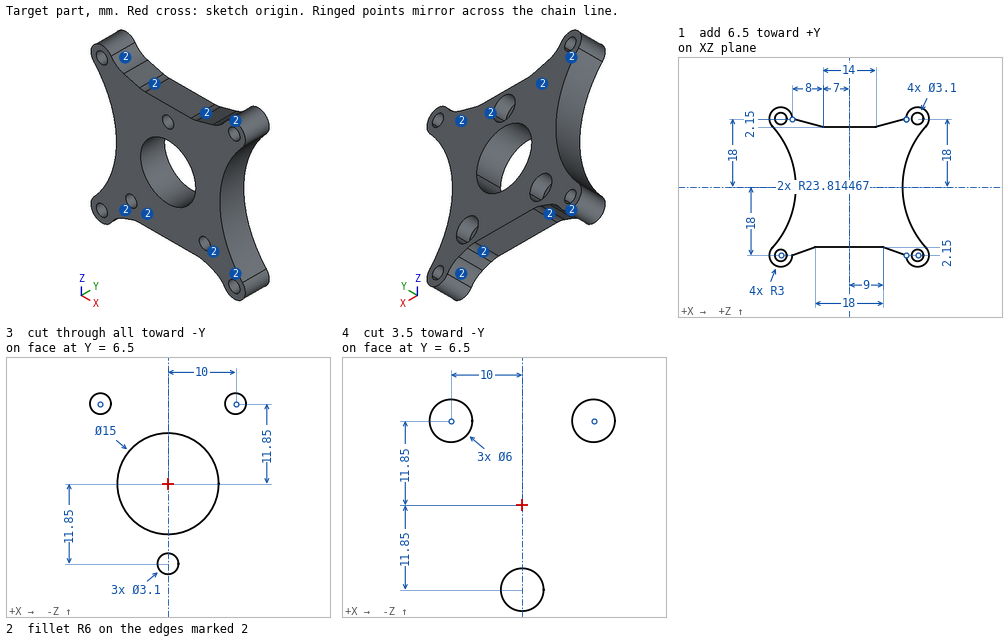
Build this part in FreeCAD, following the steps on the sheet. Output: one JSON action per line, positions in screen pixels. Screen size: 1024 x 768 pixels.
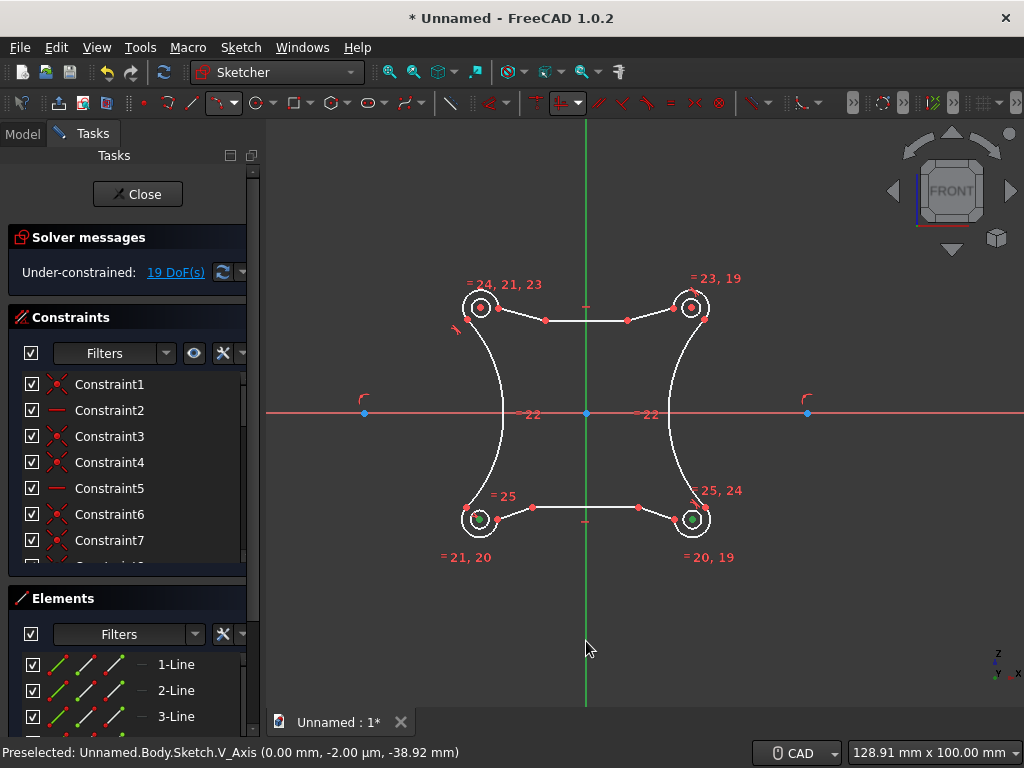
{"action": "left_click", "coordinate": [696, 104]}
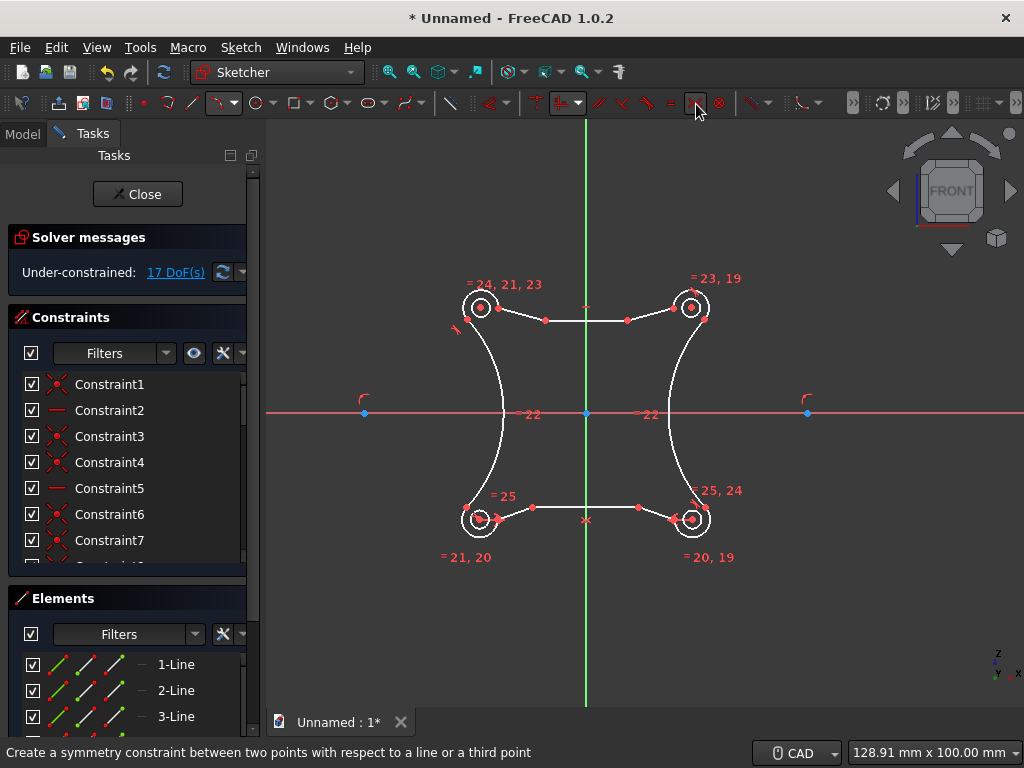
{"action": "left_click", "coordinate": [499, 308]}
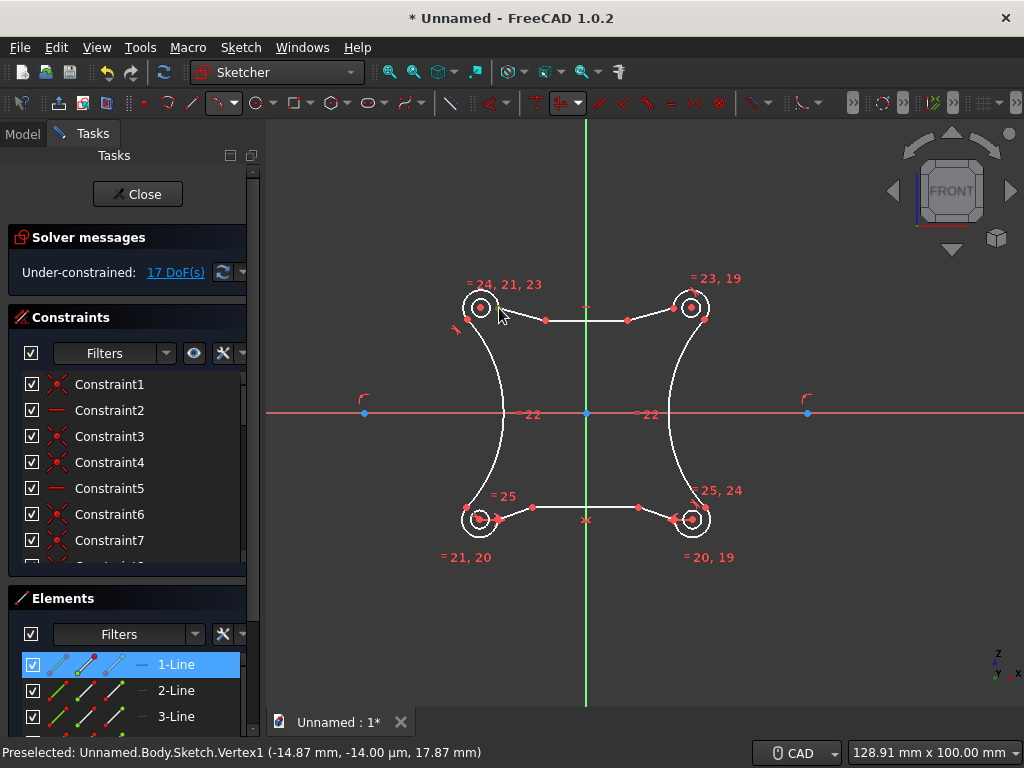
{"action": "left_click", "coordinate": [674, 308]}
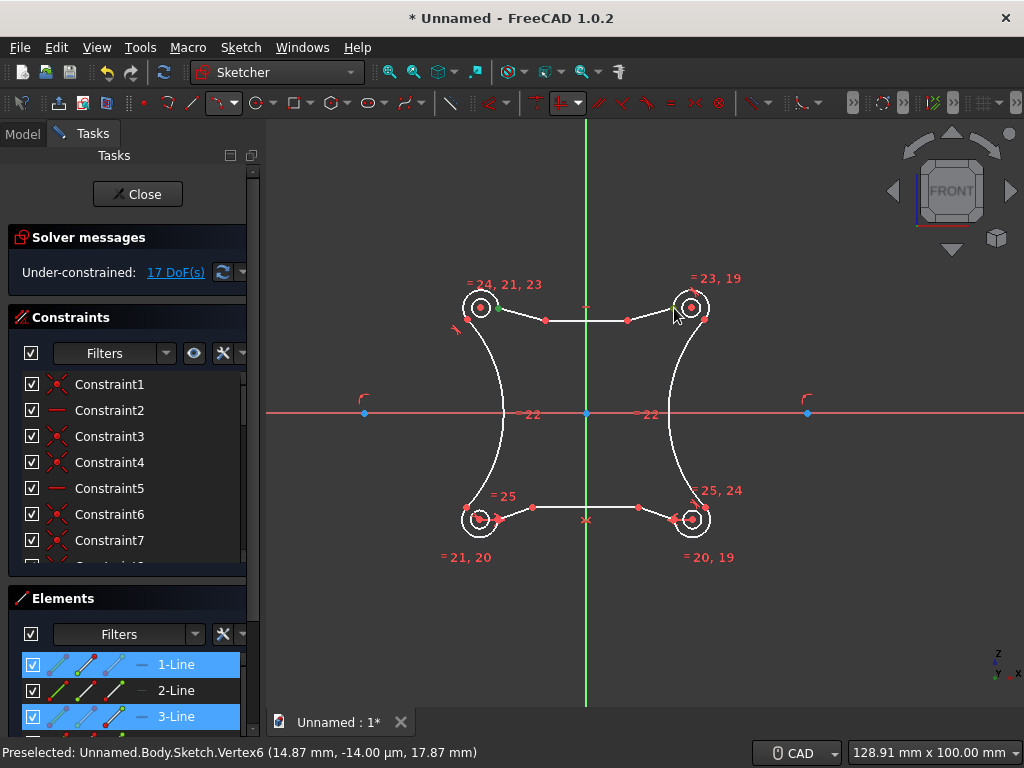
{"action": "left_click", "coordinate": [586, 641]}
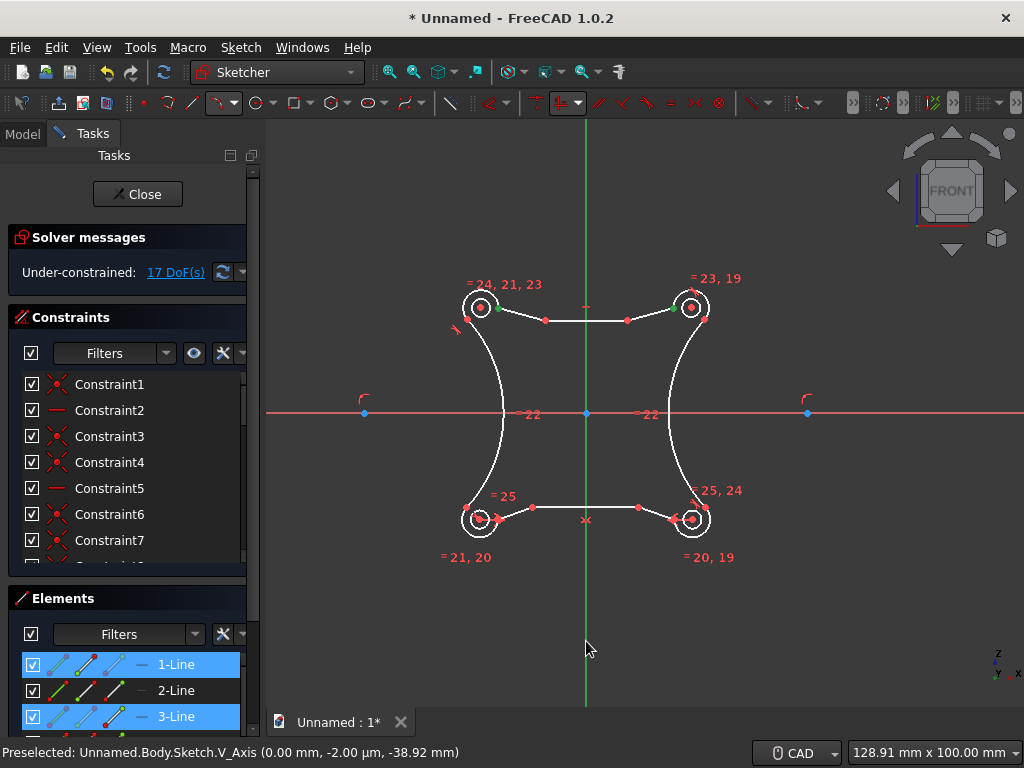
{"action": "left_click", "coordinate": [696, 104]}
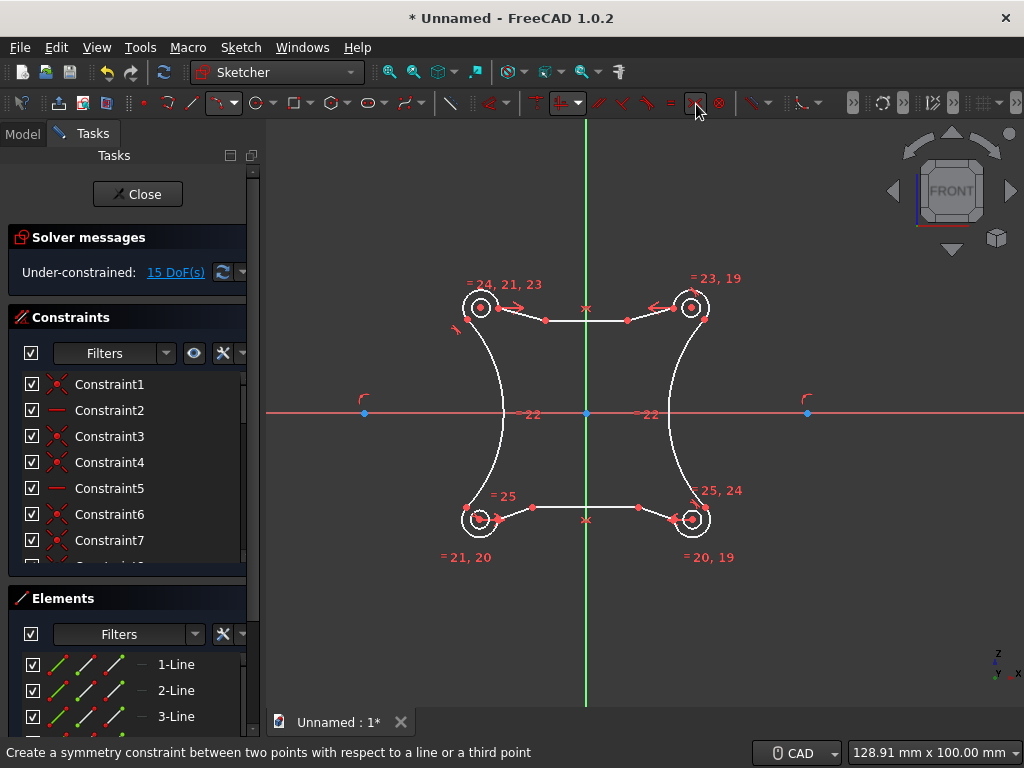
{"action": "left_click", "coordinate": [674, 308]}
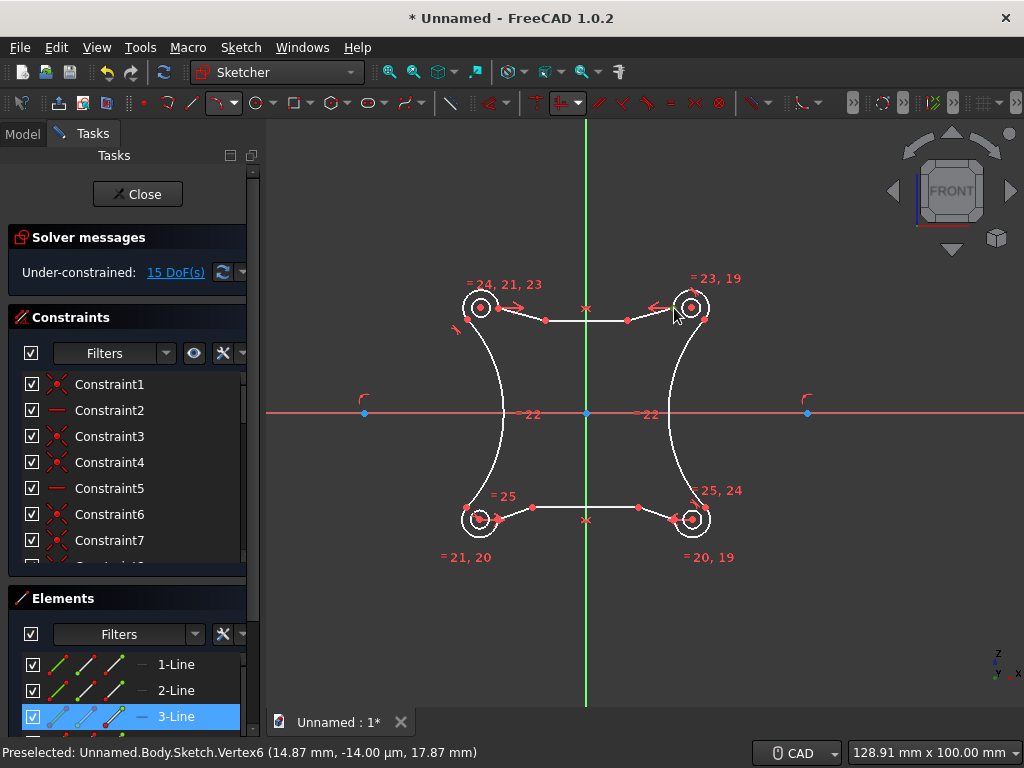
{"action": "left_click", "coordinate": [675, 520]}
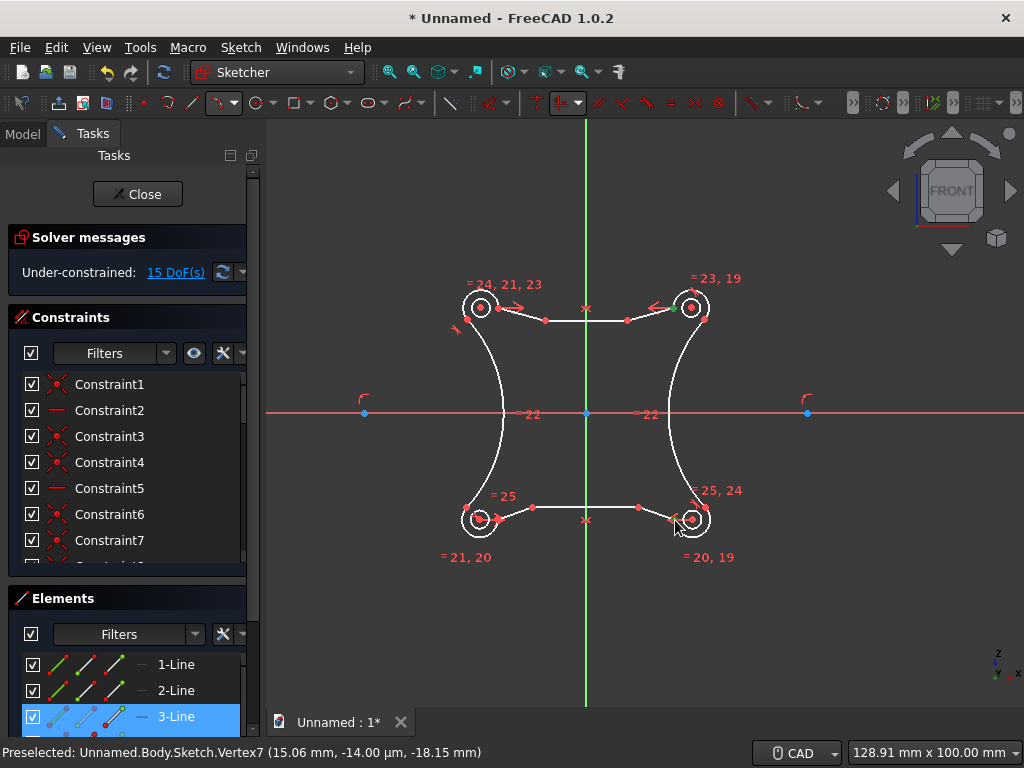
{"action": "left_click", "coordinate": [334, 413]}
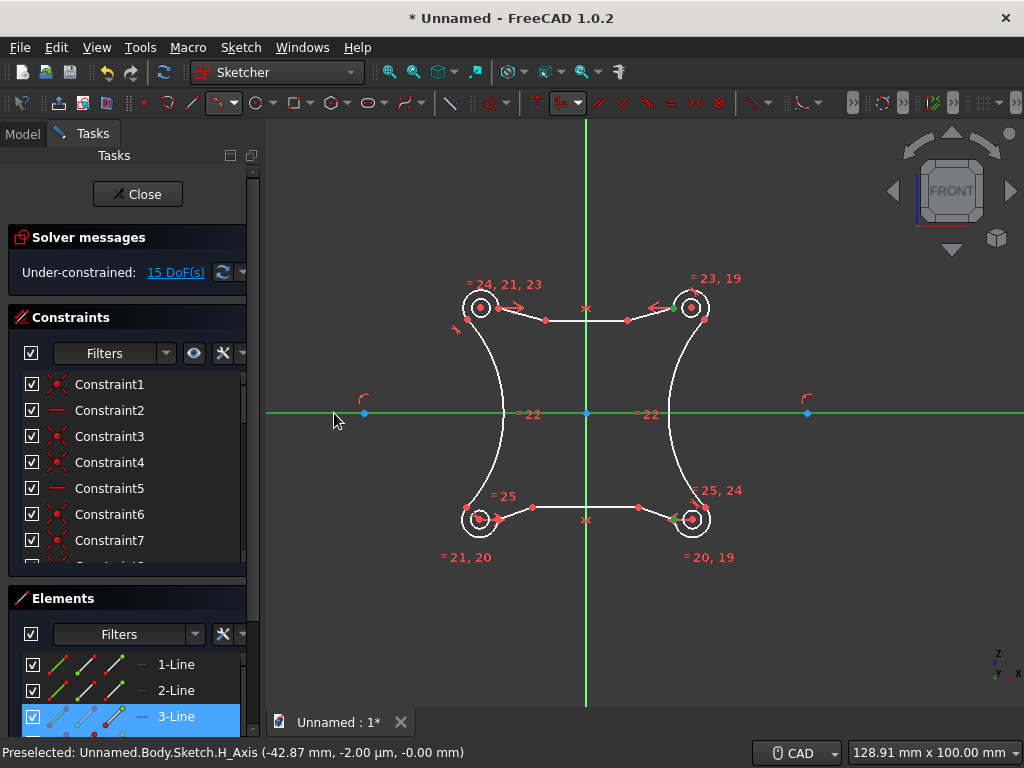
{"action": "left_click", "coordinate": [696, 104]}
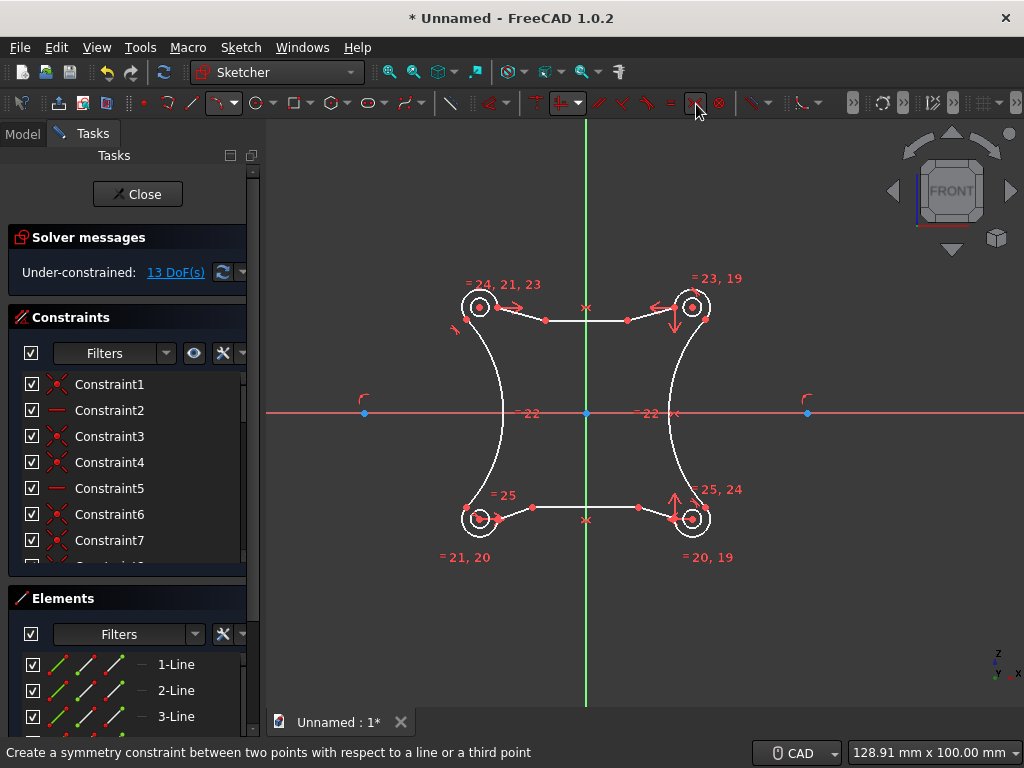
{"action": "scroll", "coordinate": [708, 300], "scroll_direction": "up", "scroll_amount": 5}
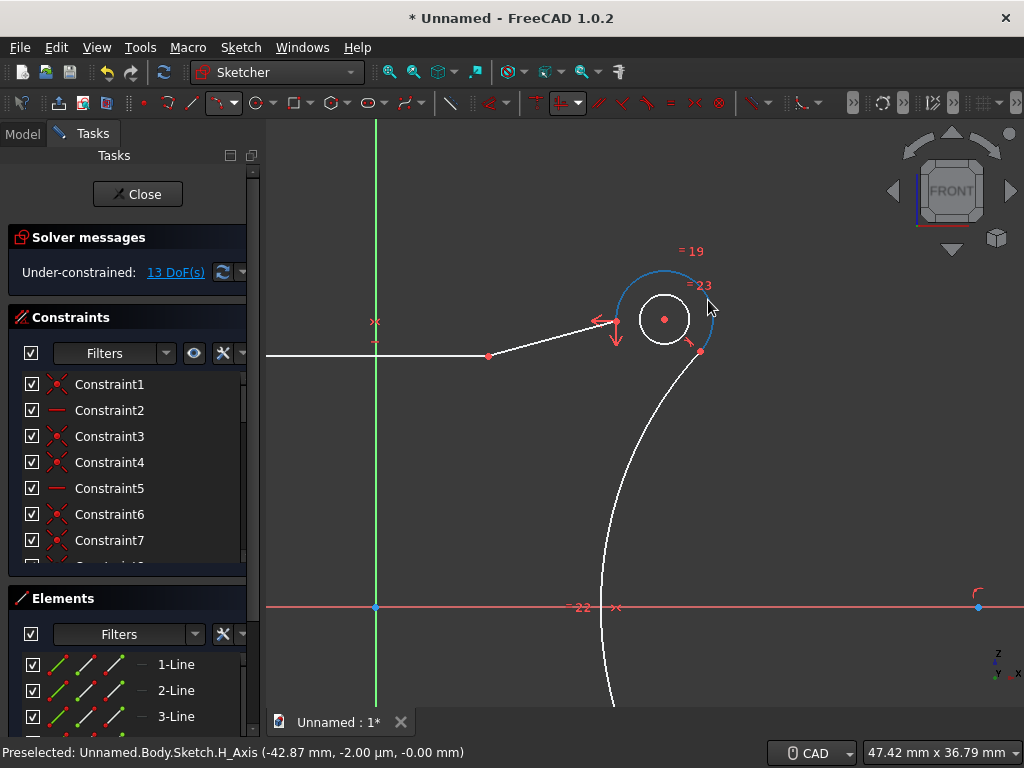
{"action": "left_click", "coordinate": [708, 299]}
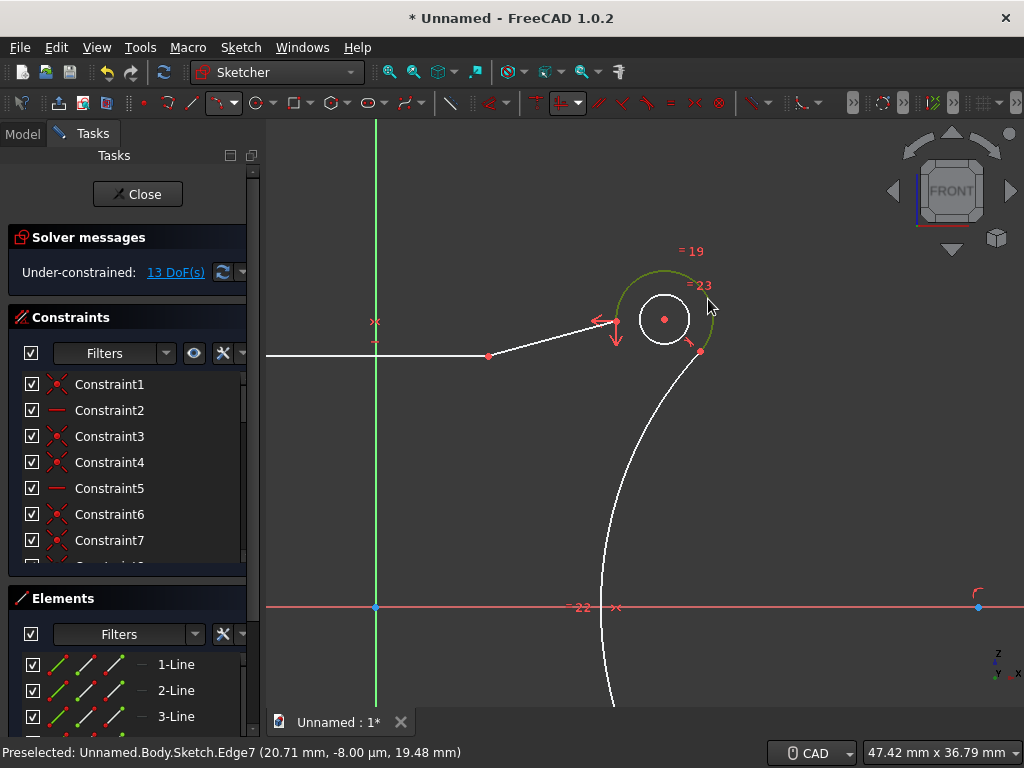
{"action": "key", "text": "k r"}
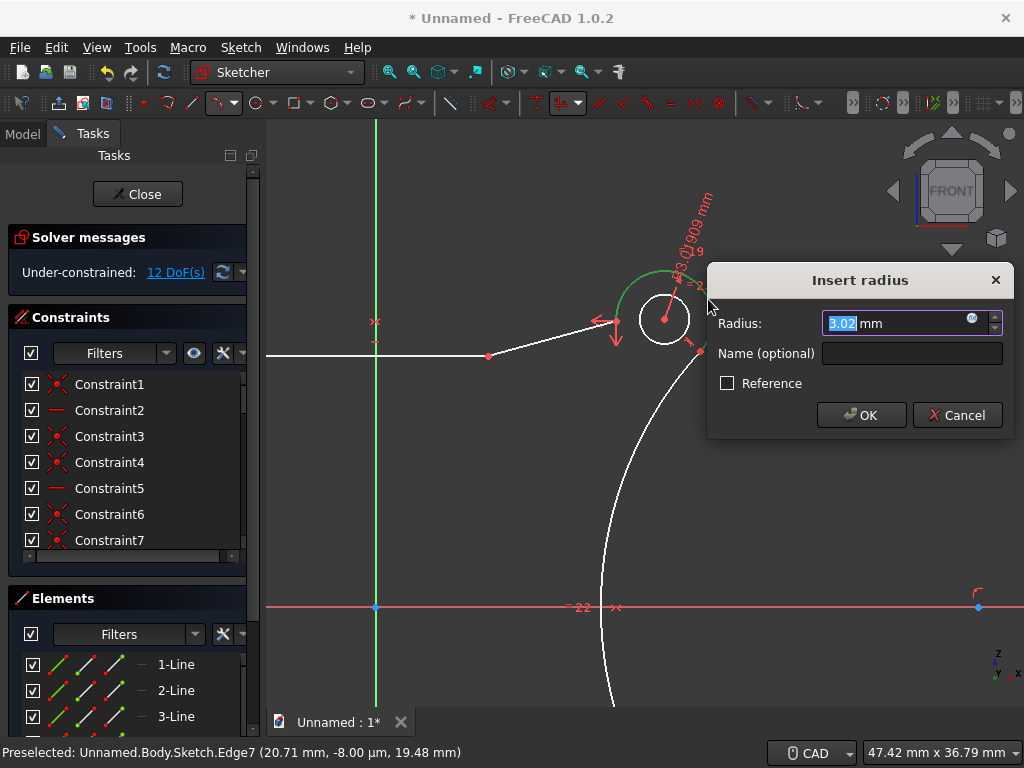
{"action": "type", "text": "3"}
{"action": "key", "text": "Return"}